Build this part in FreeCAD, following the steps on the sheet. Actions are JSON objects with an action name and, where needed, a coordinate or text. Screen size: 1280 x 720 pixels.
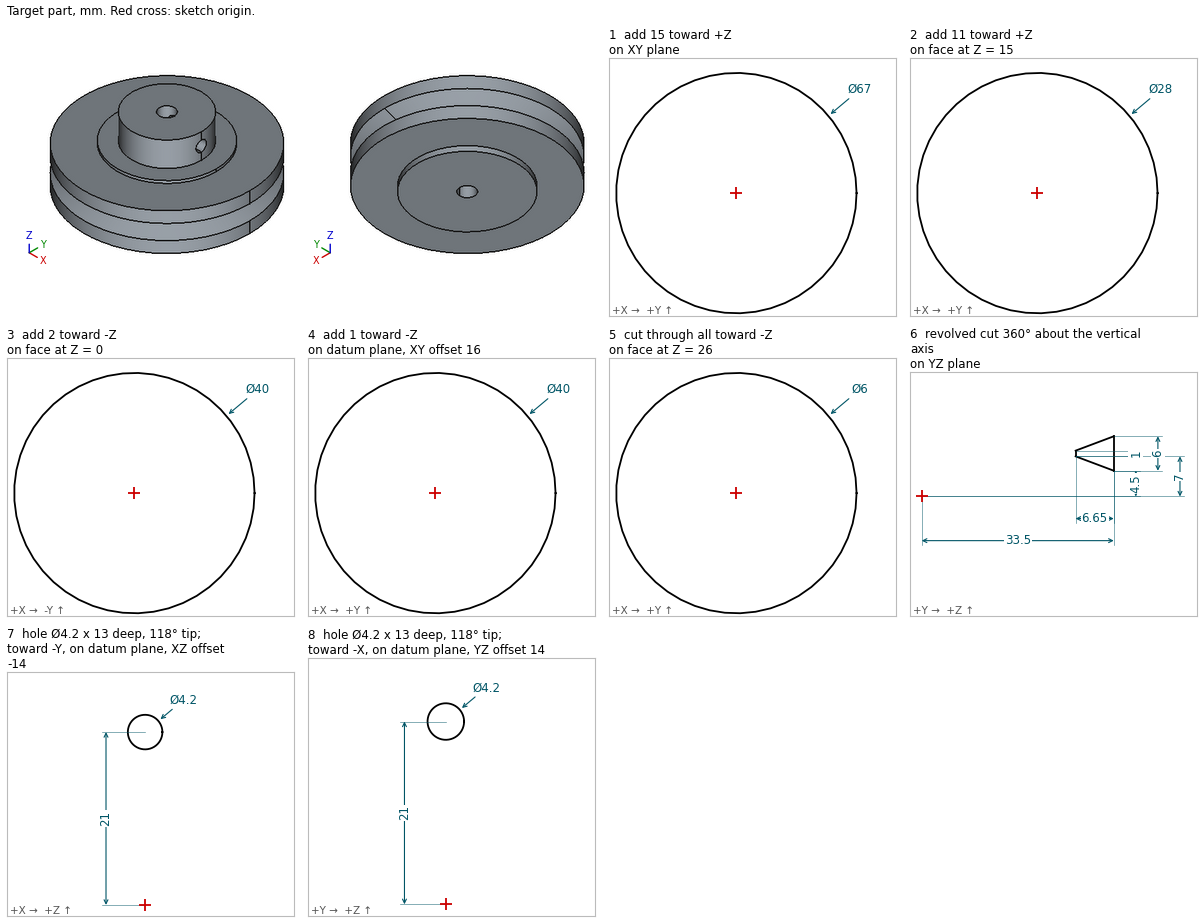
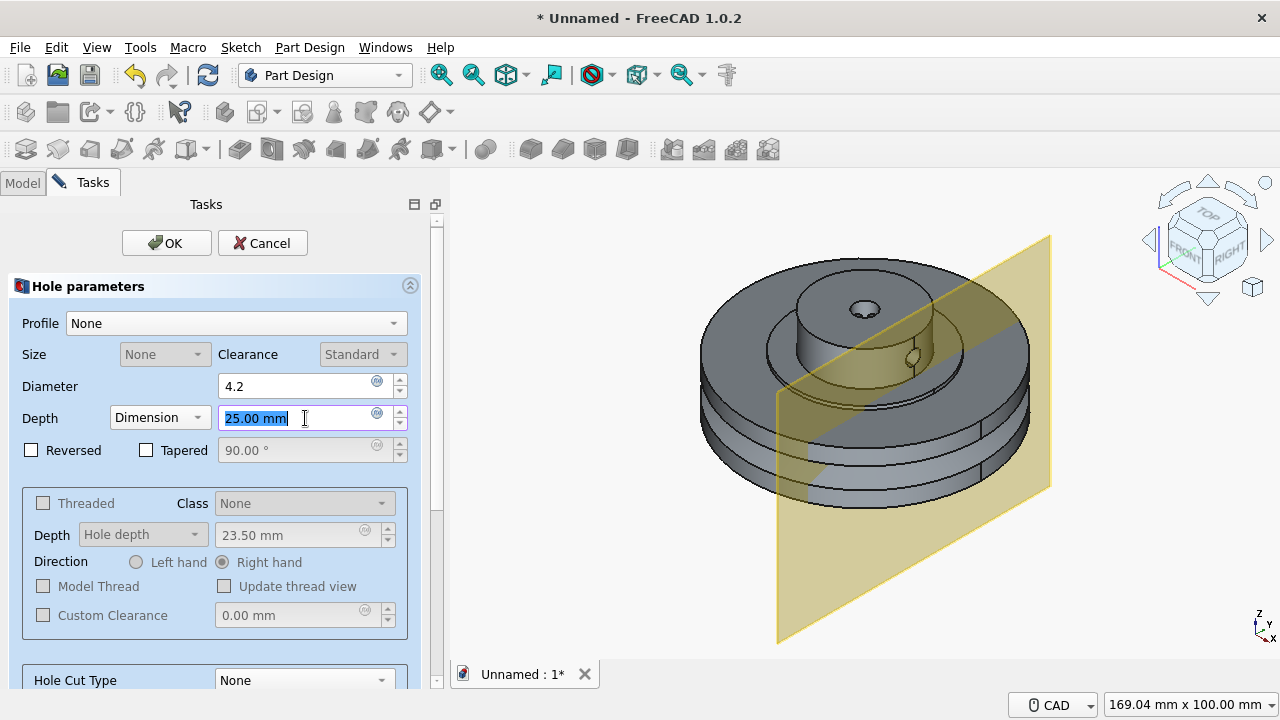
{"action": "type", "text": "13"}
{"action": "key", "text": "Tab"}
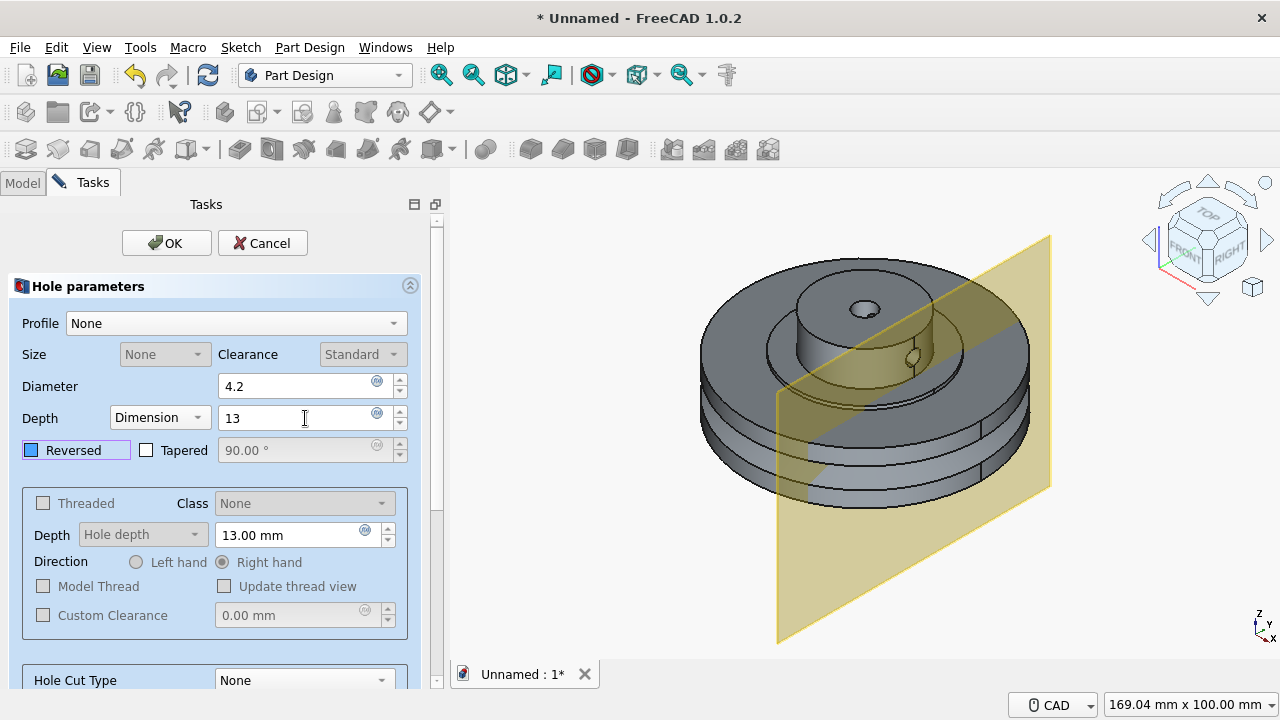
{"action": "left_click", "coordinate": [167, 243]}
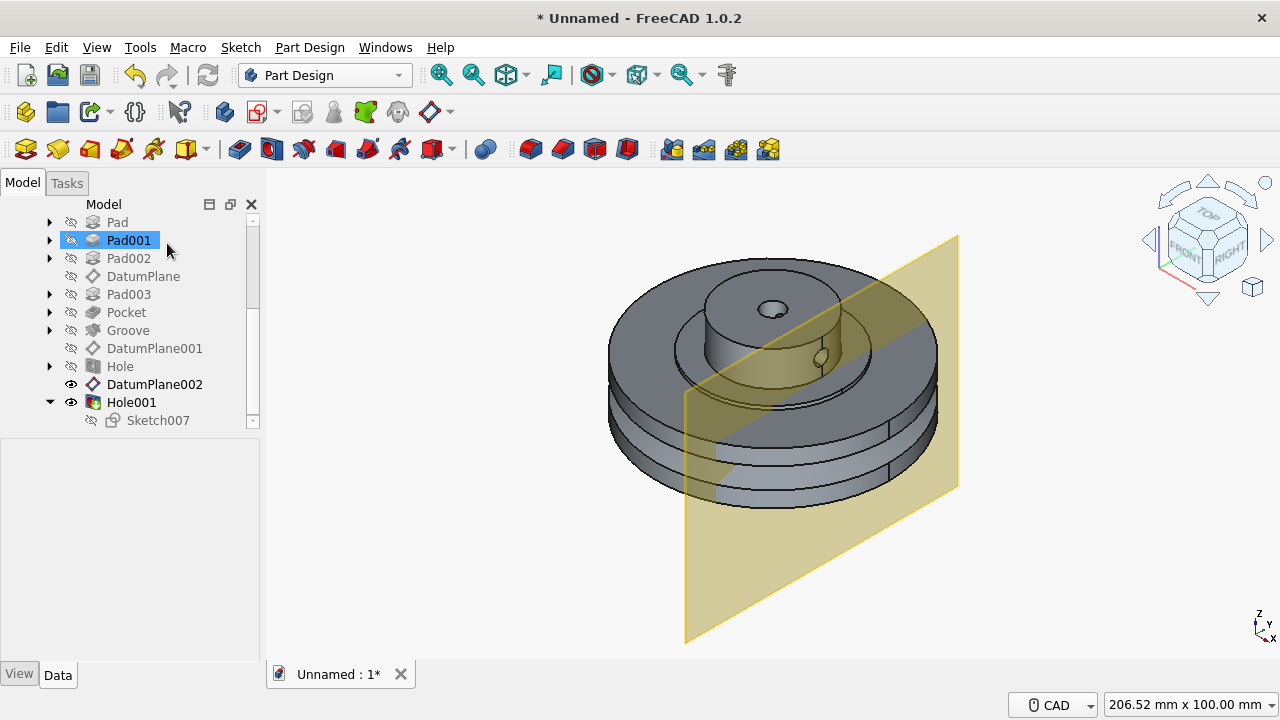
{"action": "left_click", "coordinate": [116, 384]}
{"action": "key", "text": "space"}